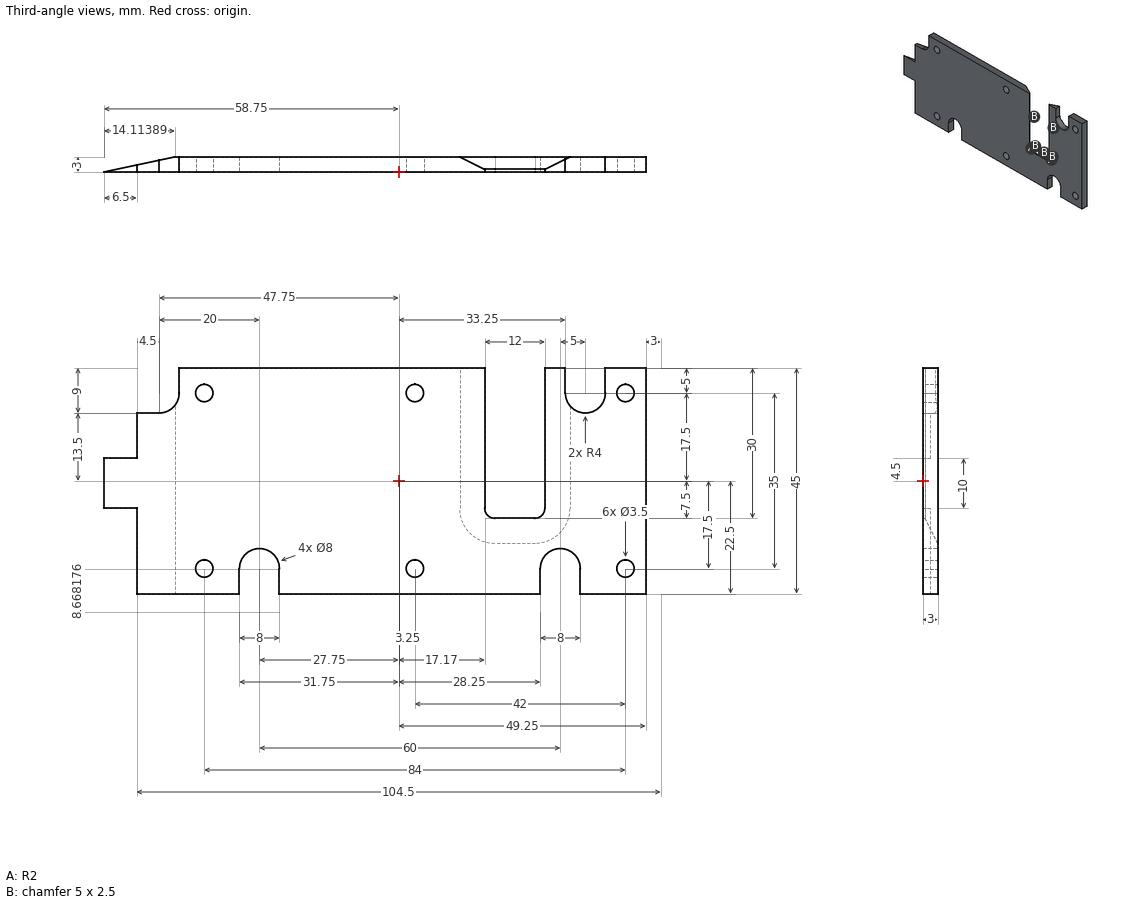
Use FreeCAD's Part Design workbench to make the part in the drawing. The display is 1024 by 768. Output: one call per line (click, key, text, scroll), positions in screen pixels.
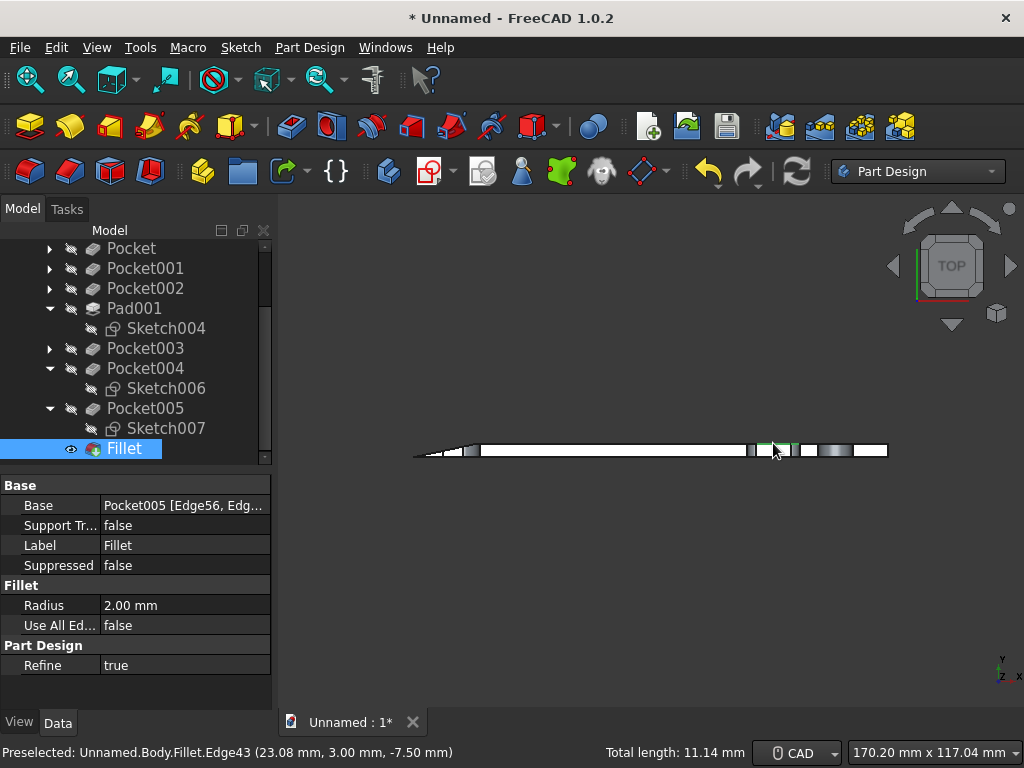
click(754, 443, ctrl)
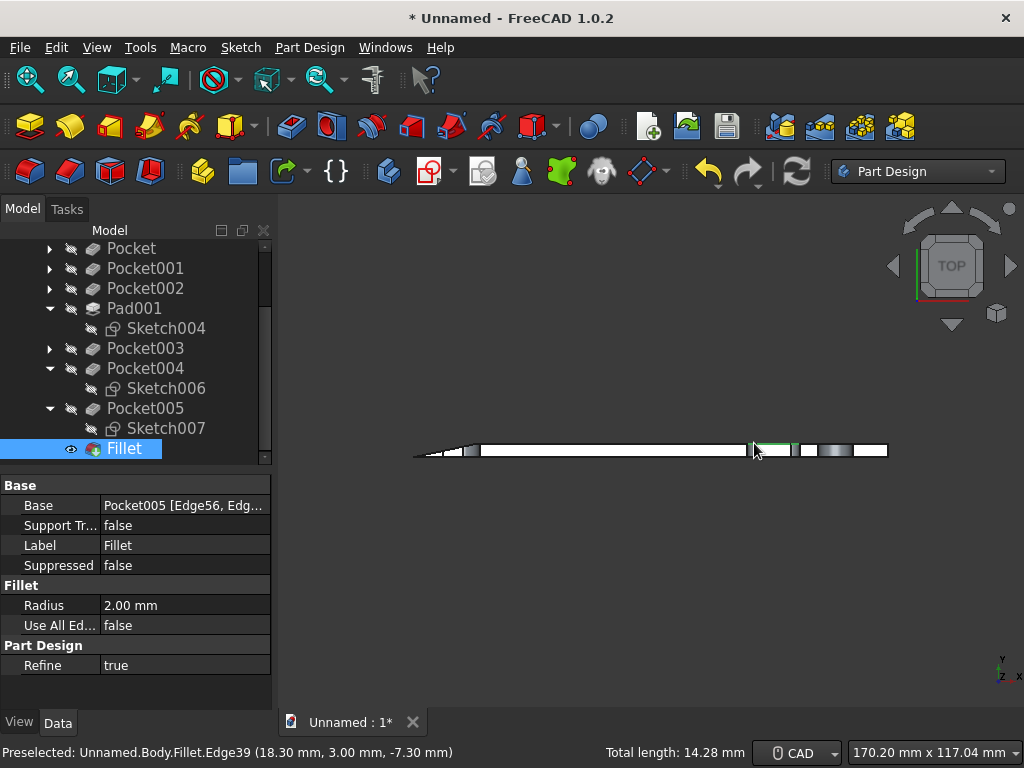
key(0)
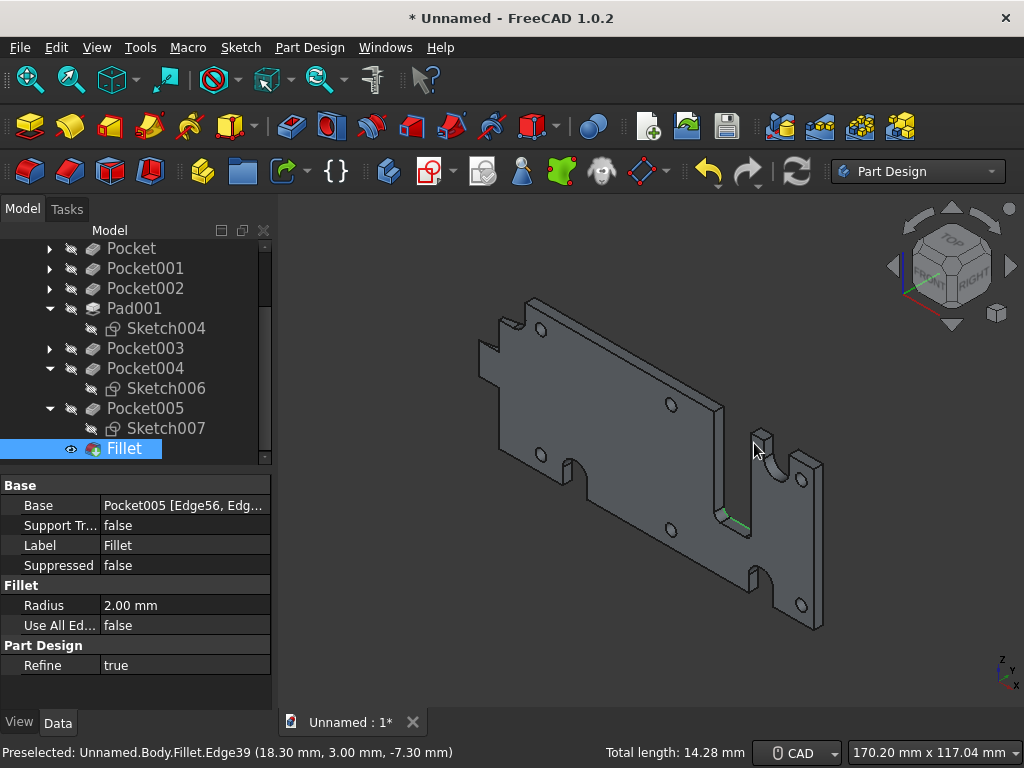
key(1)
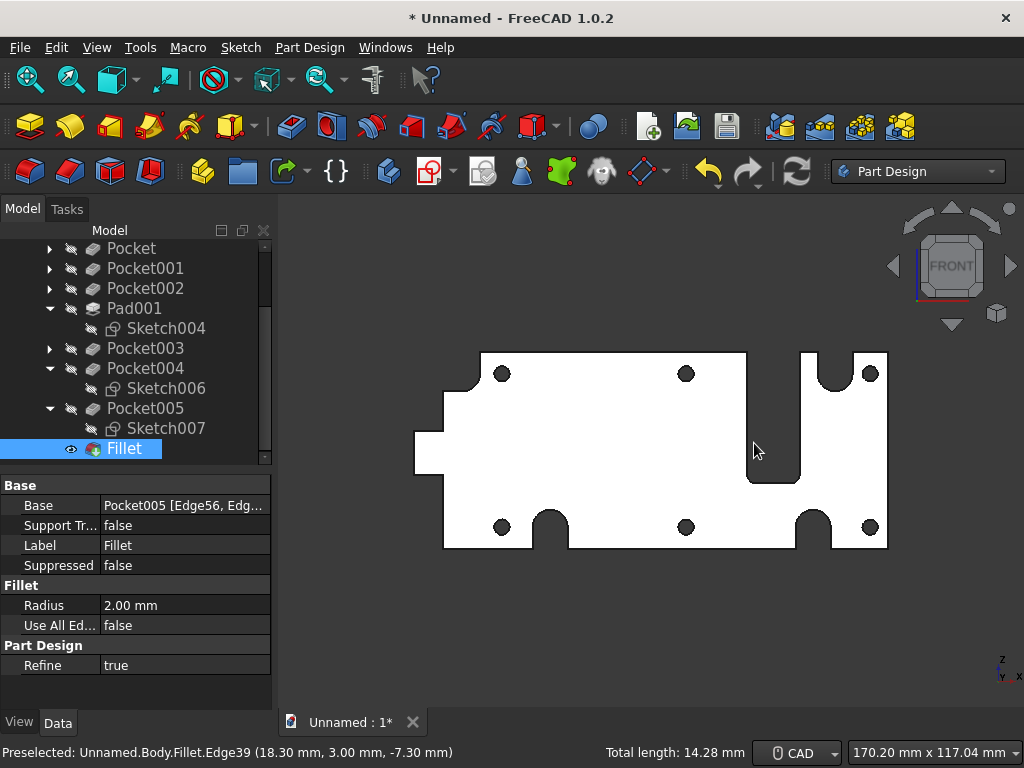
key(3)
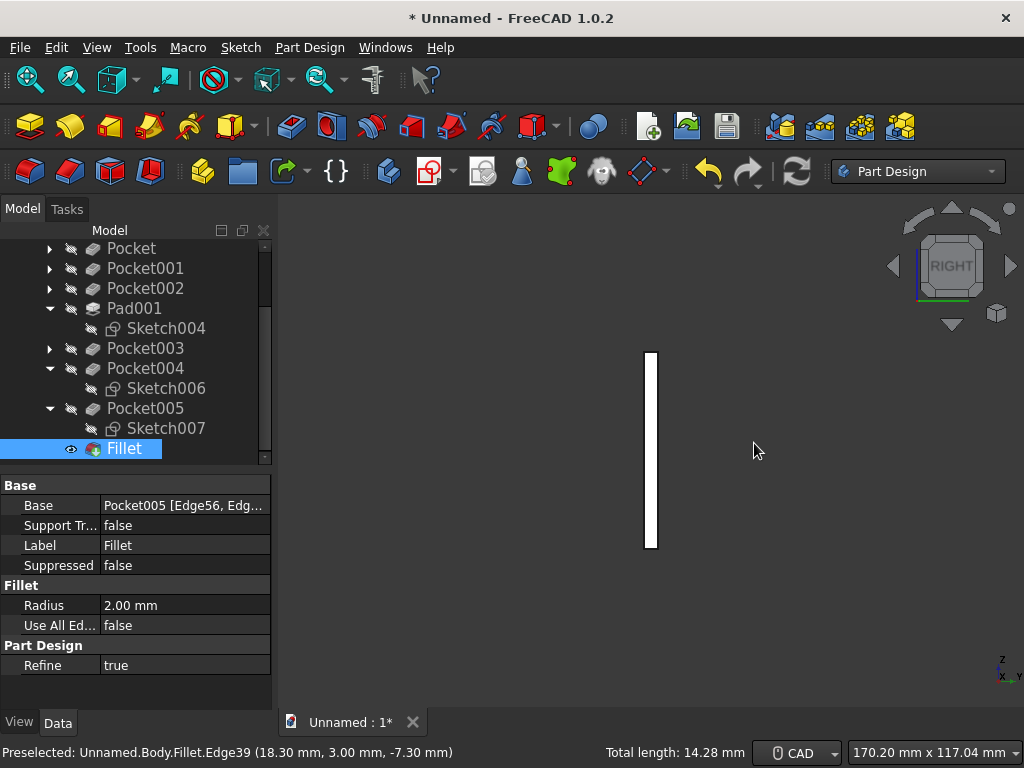
key(v)
key(f)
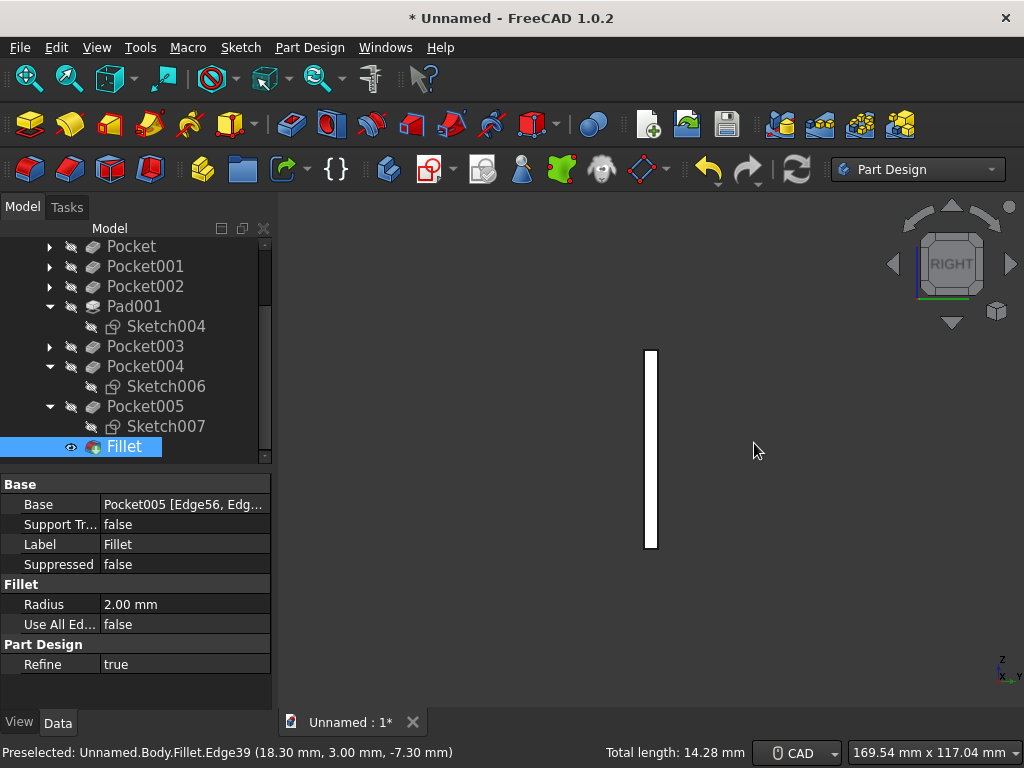
key(5)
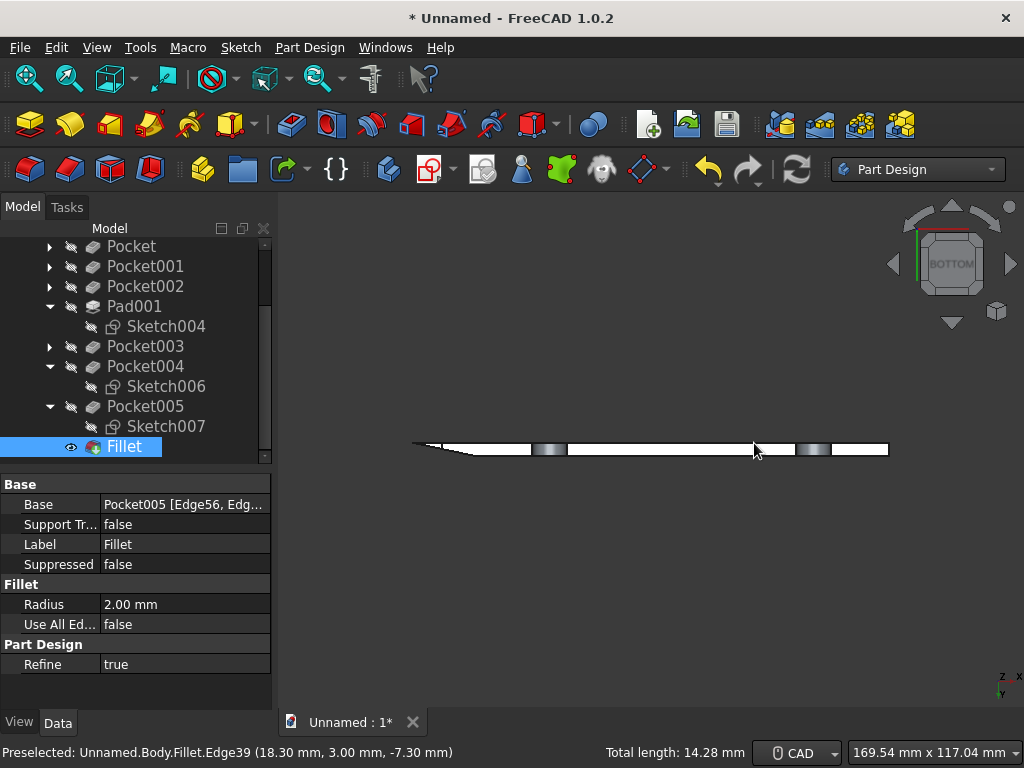
key(4)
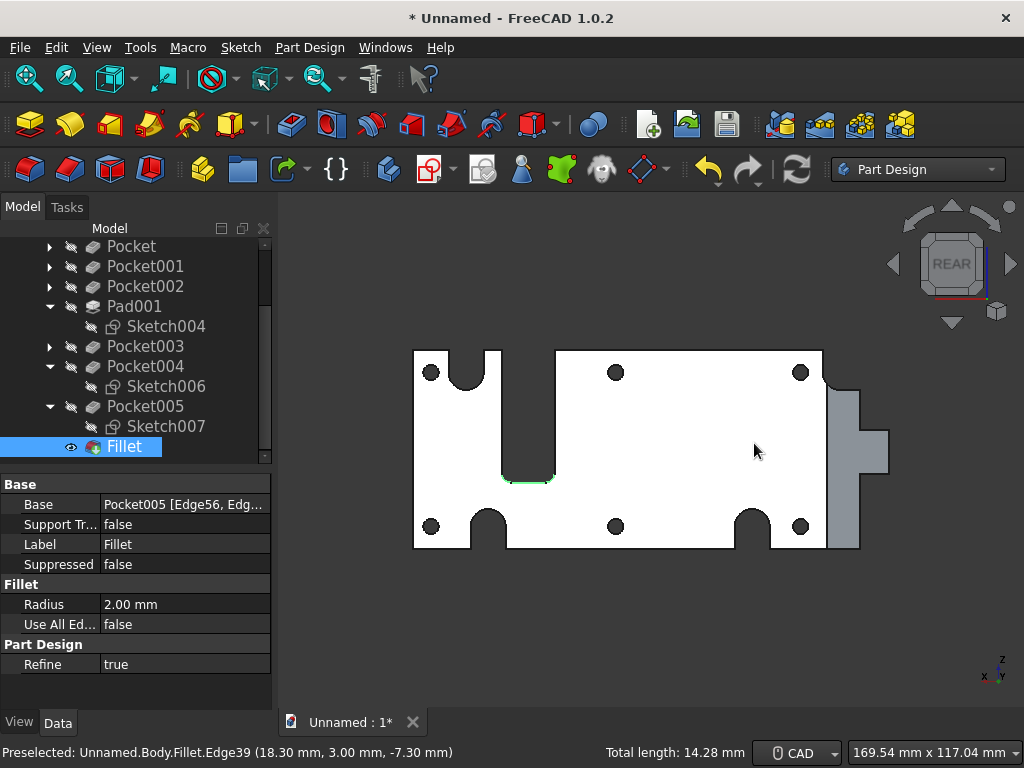
click(502, 411, ctrl)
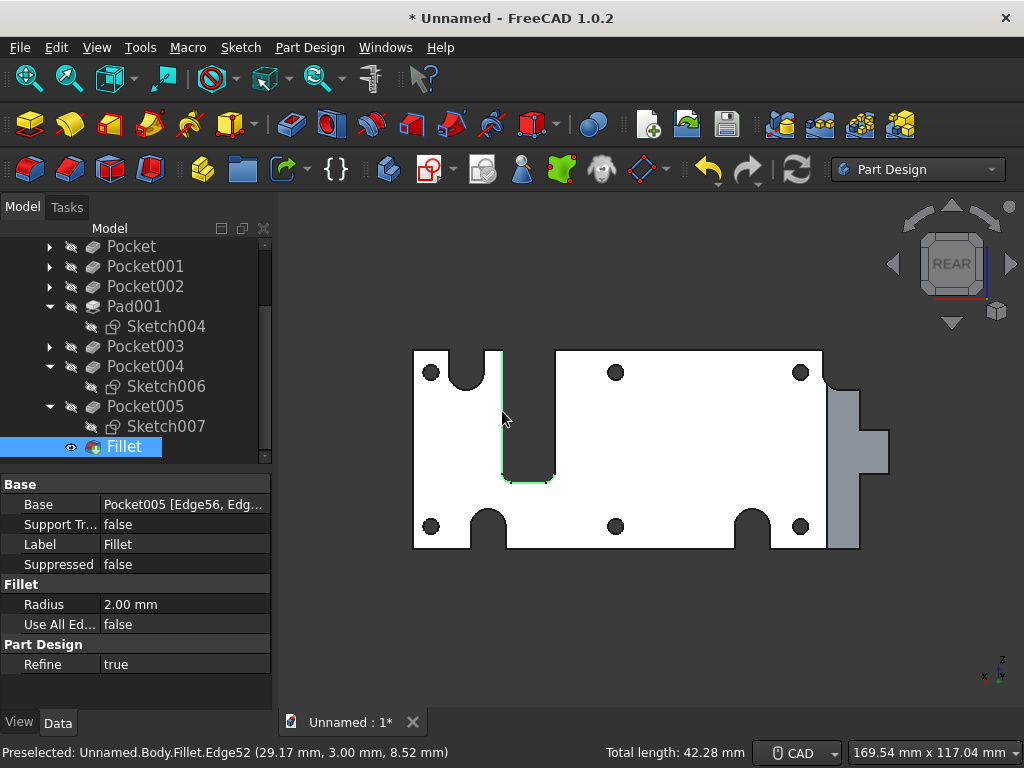
click(555, 411, ctrl)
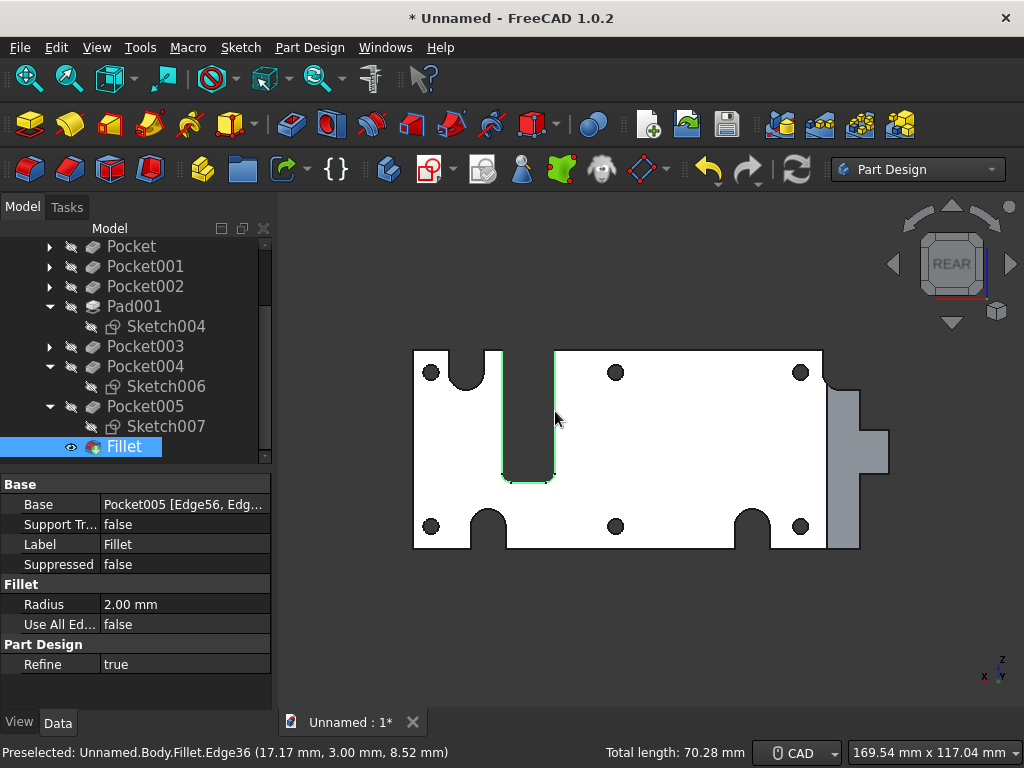
click(70, 170)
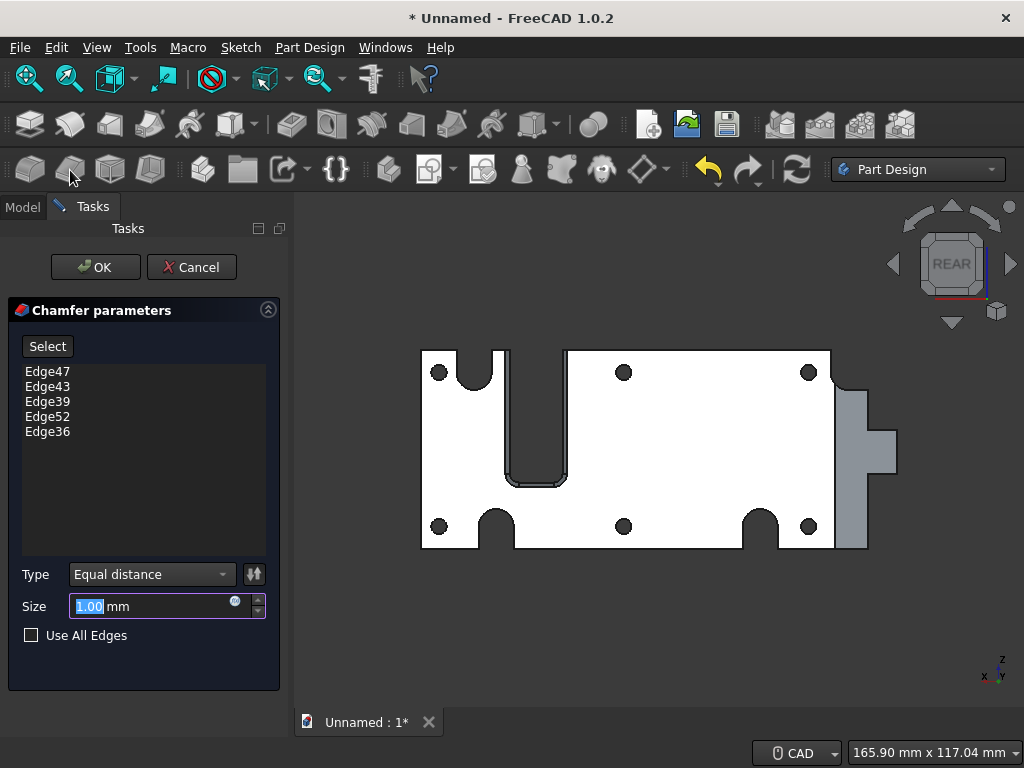
text(5)
key(Tab)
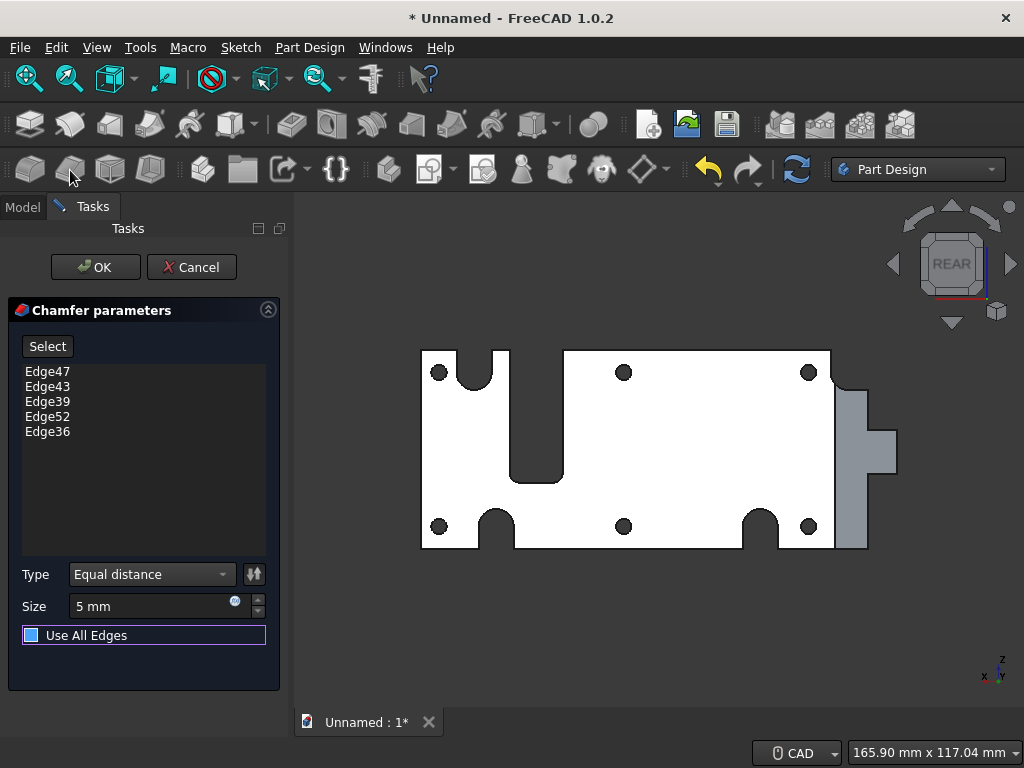
click(153, 574)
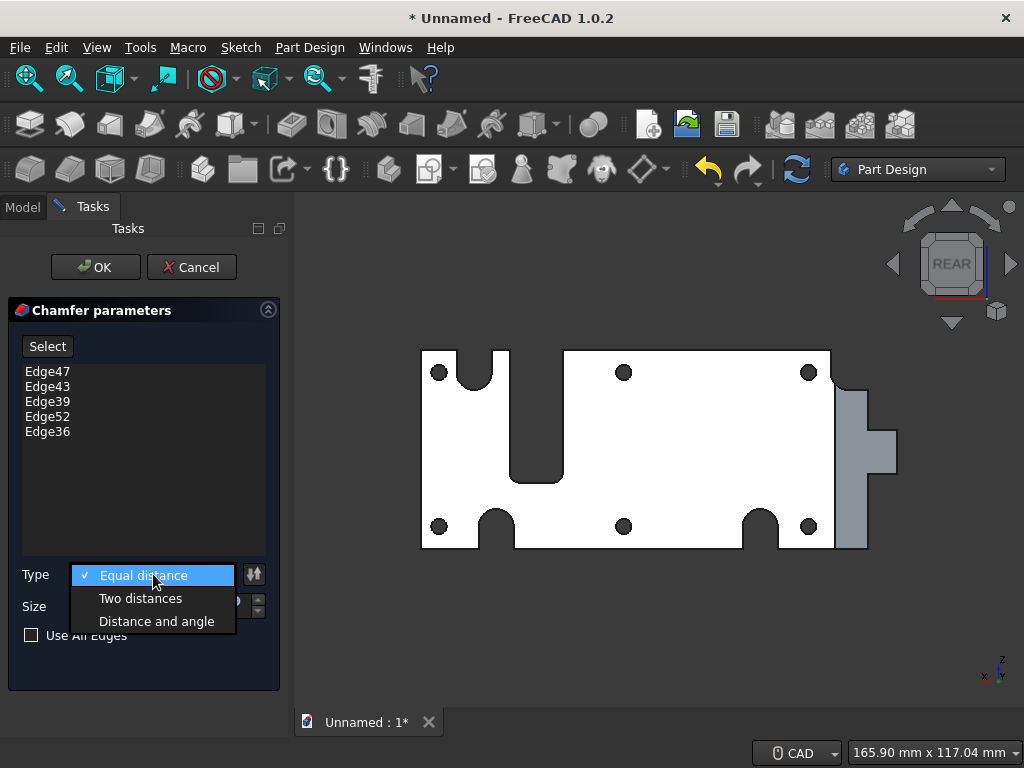
click(152, 598)